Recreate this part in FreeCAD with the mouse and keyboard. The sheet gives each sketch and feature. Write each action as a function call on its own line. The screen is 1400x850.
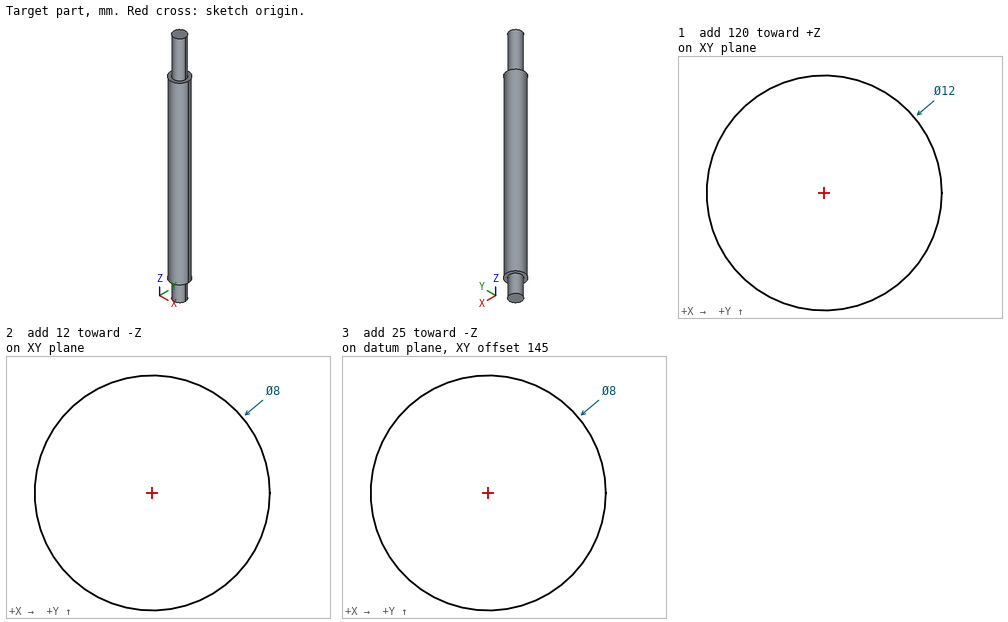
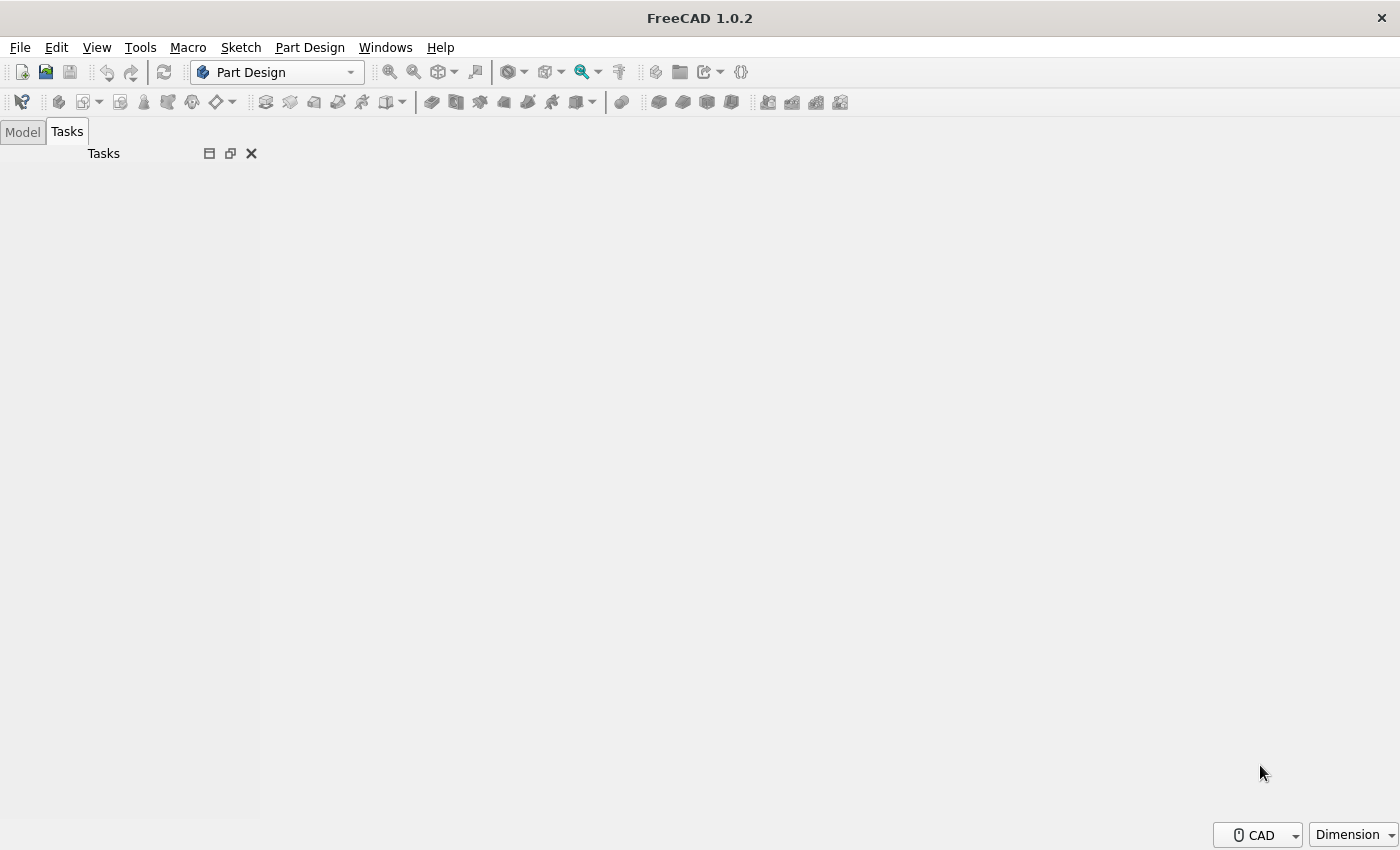
click(22, 72)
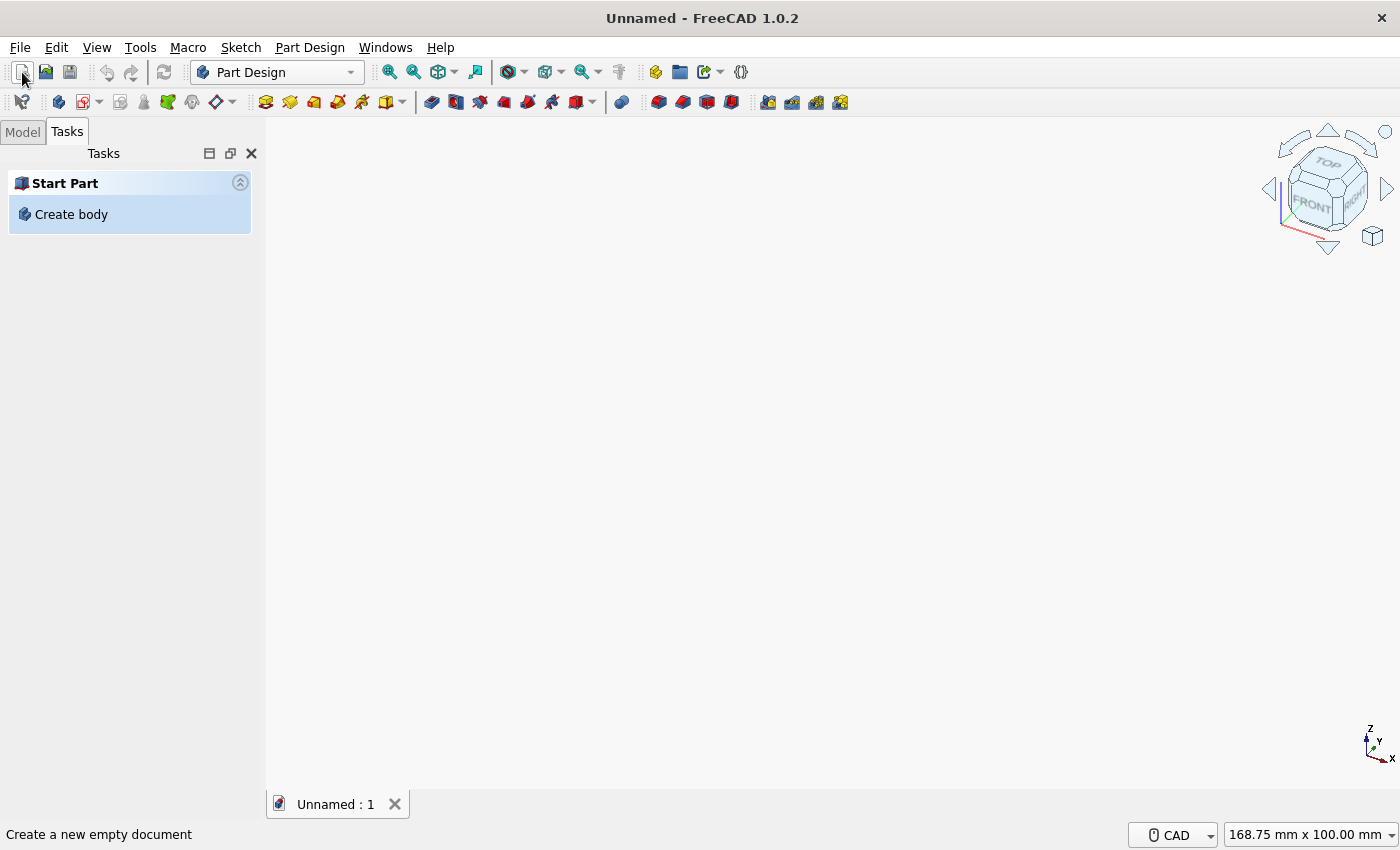
click(84, 102)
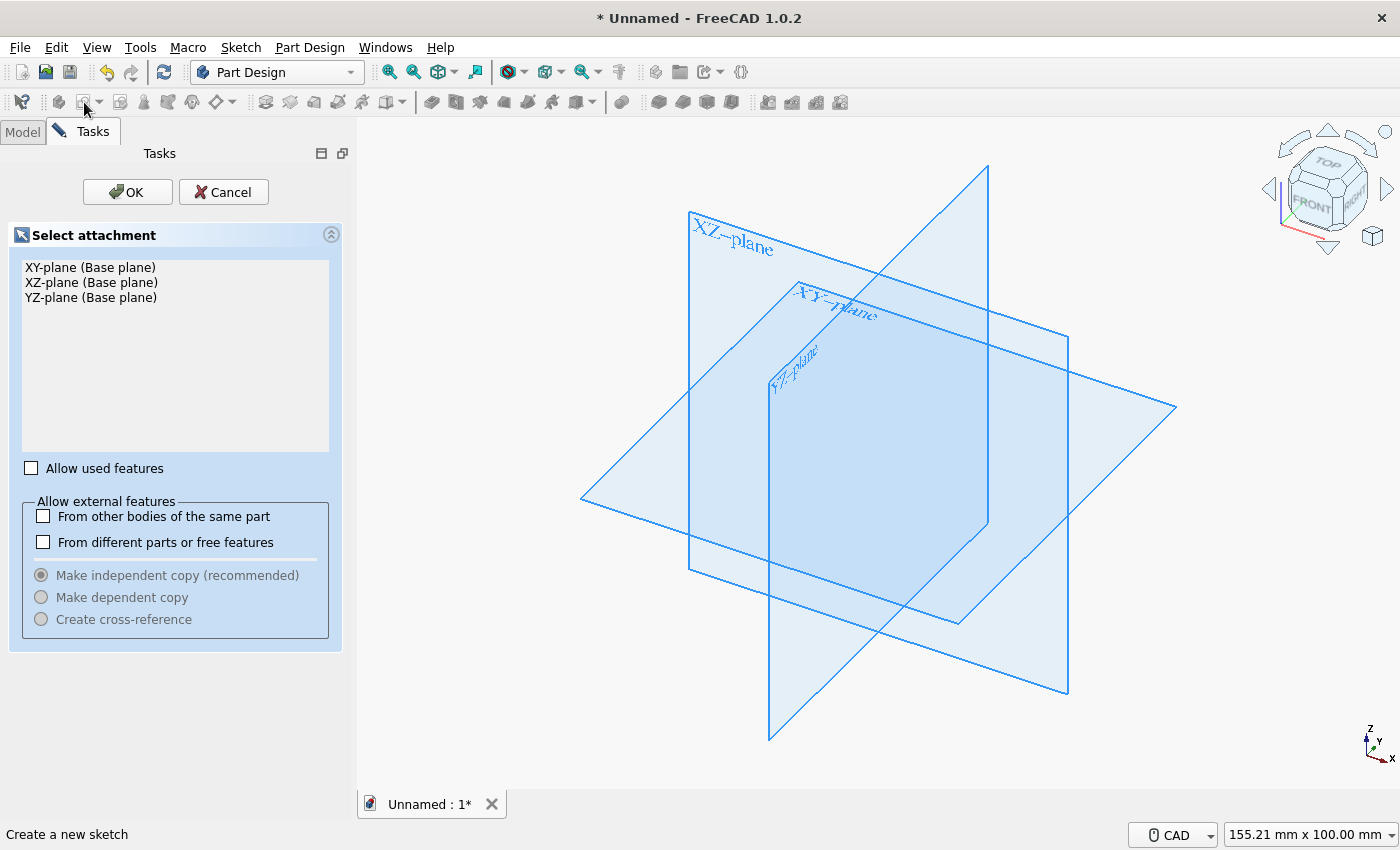
click(82, 268)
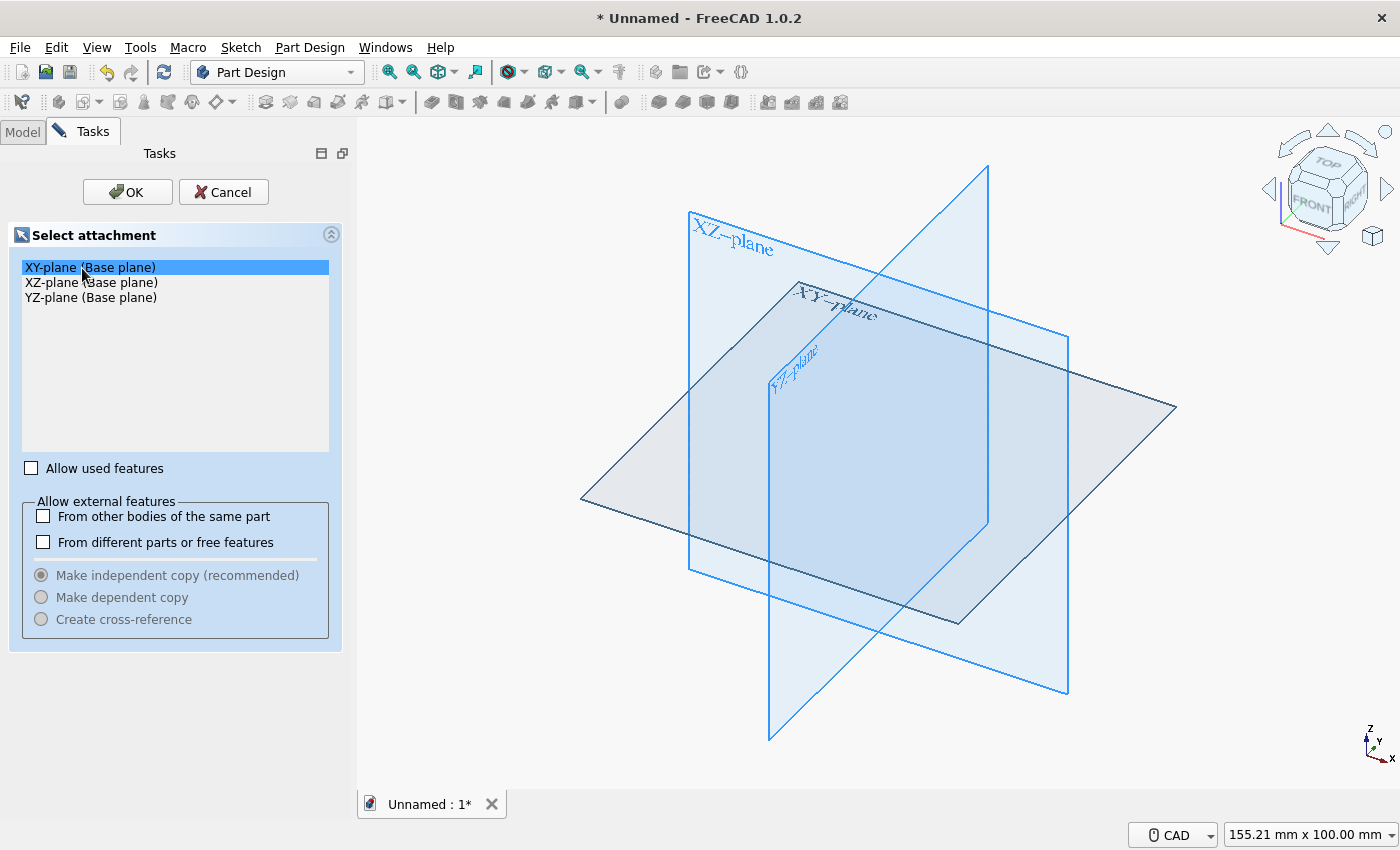
click(128, 192)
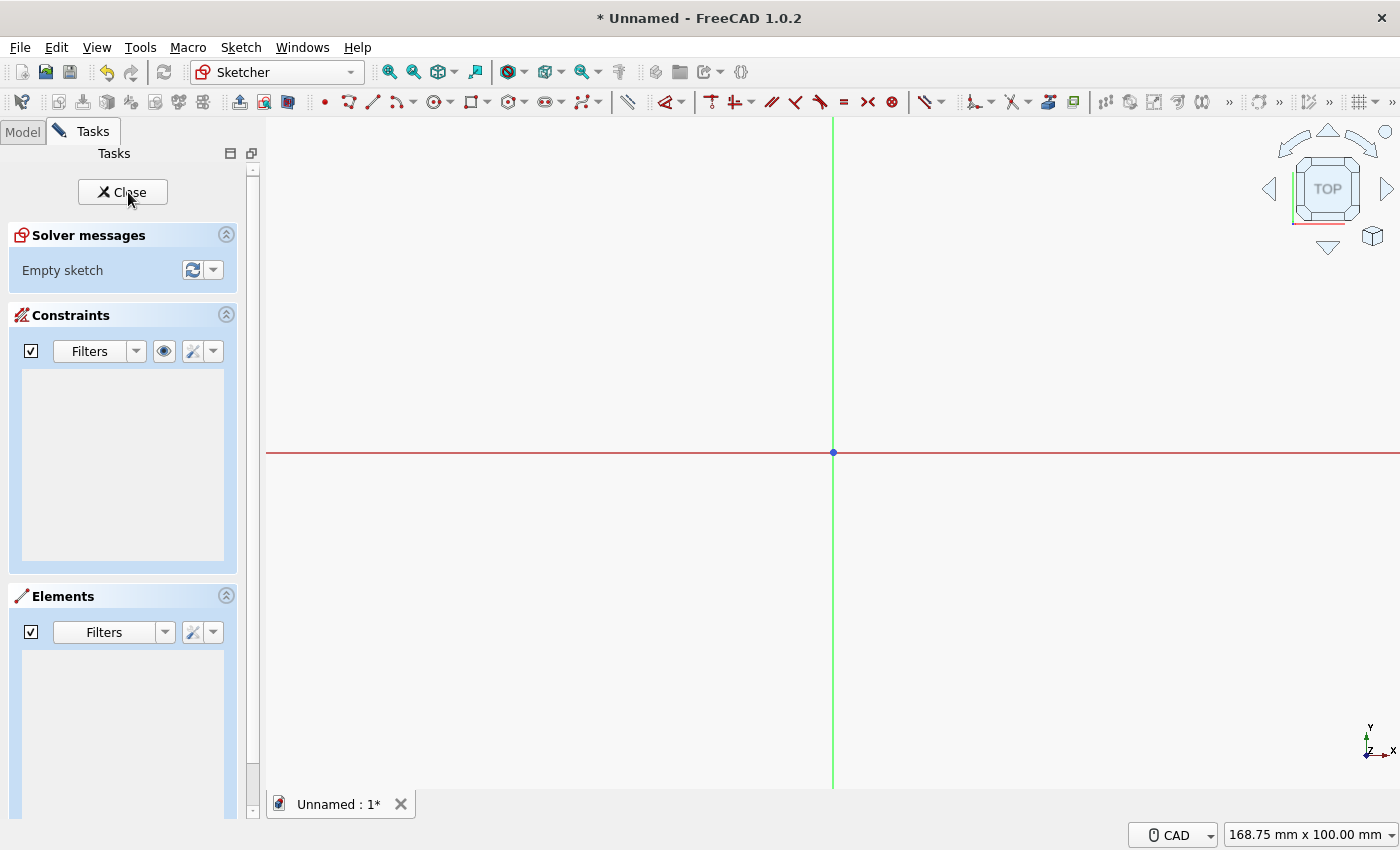
scroll(850, 453, up, 8)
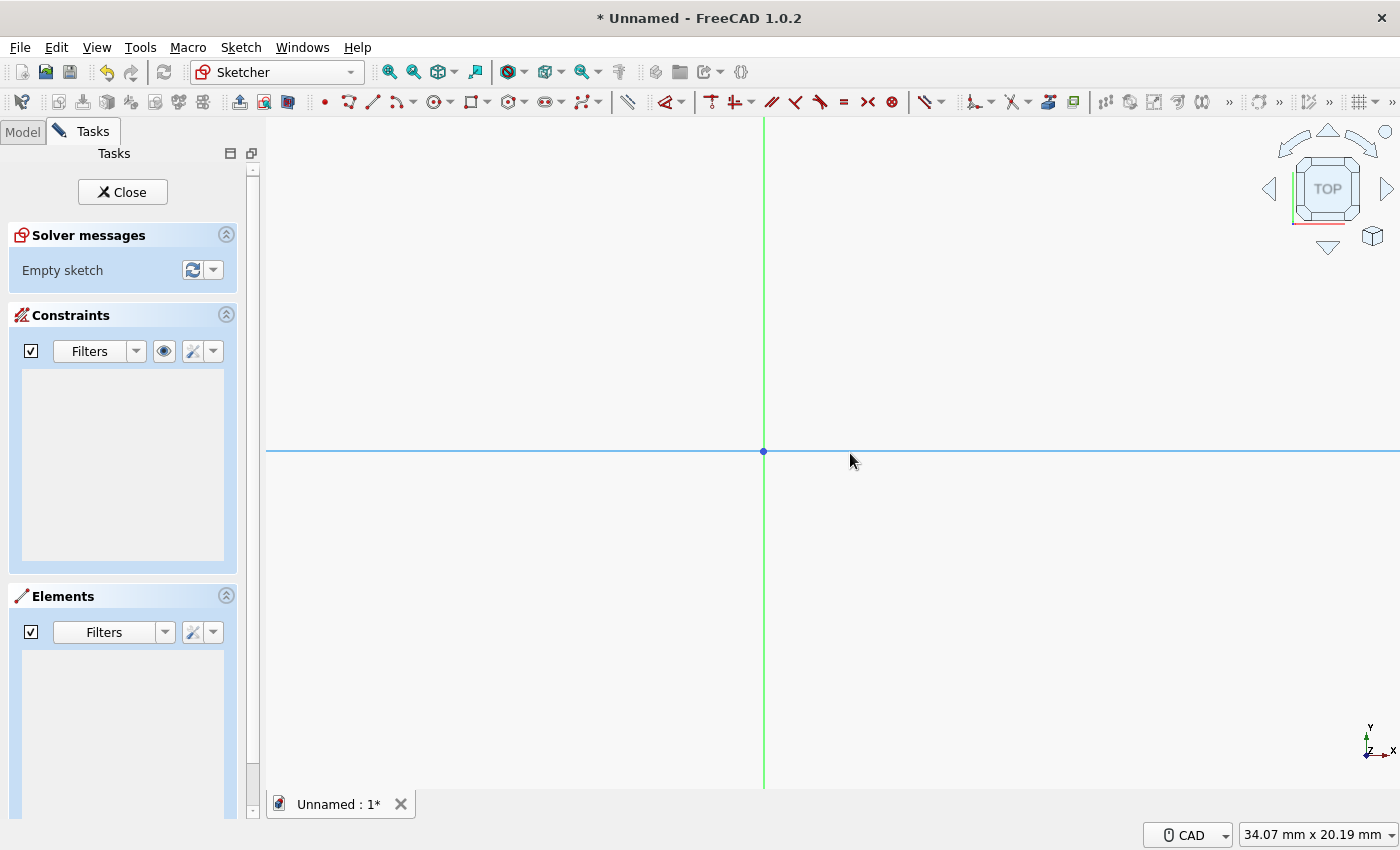
key(g)
key(c)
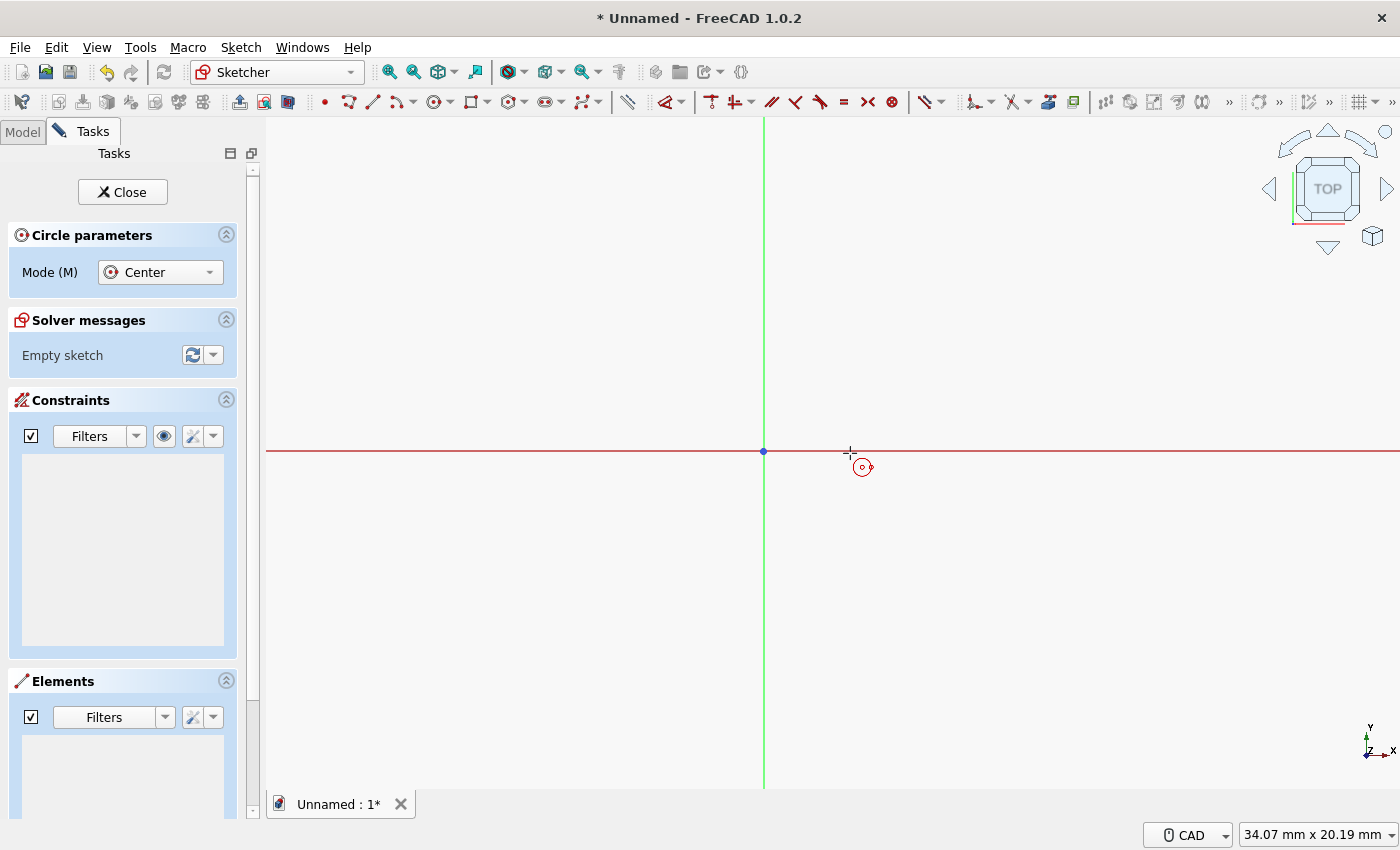
click(764, 451)
click(905, 310)
key(Escape)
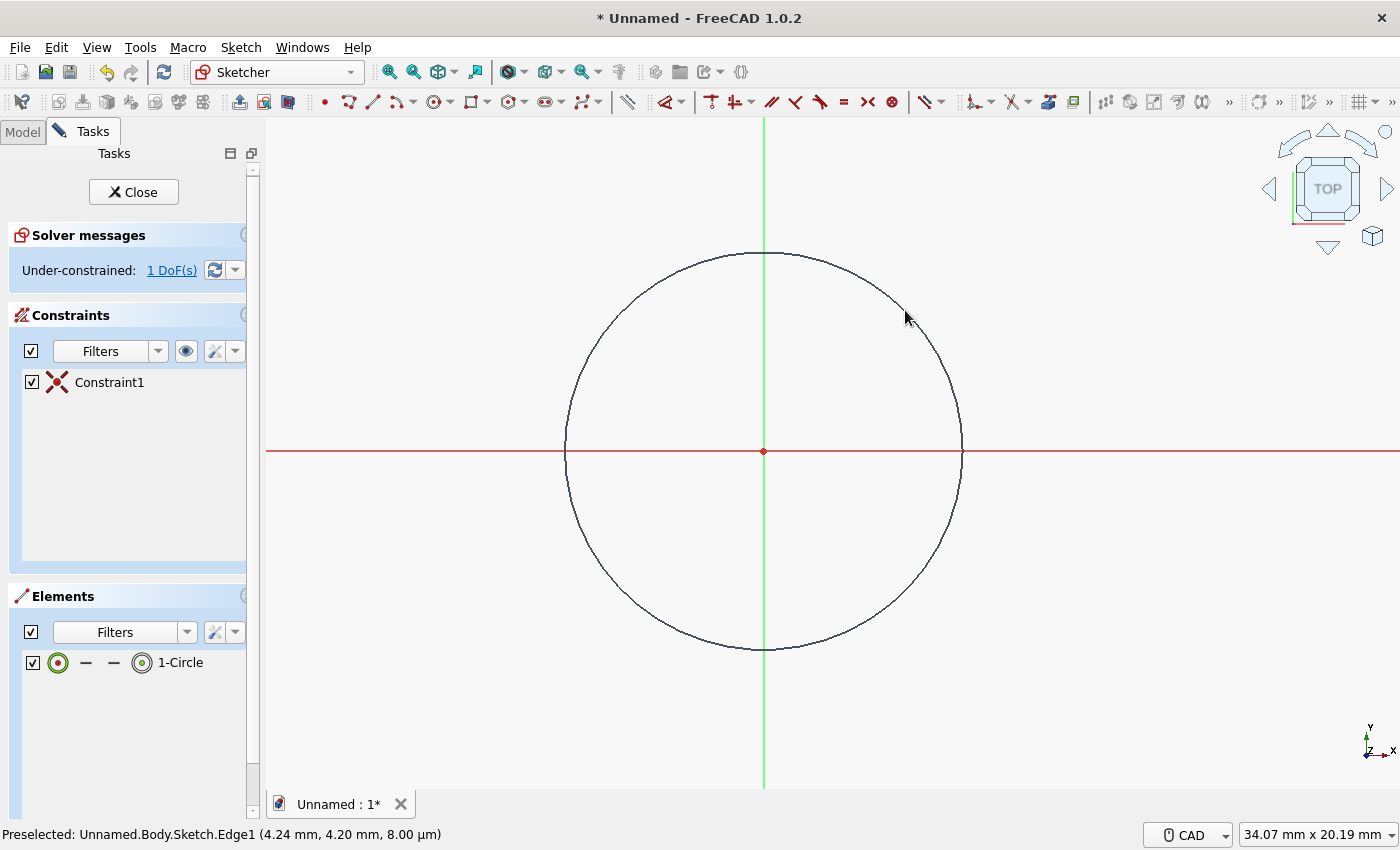
click(666, 102)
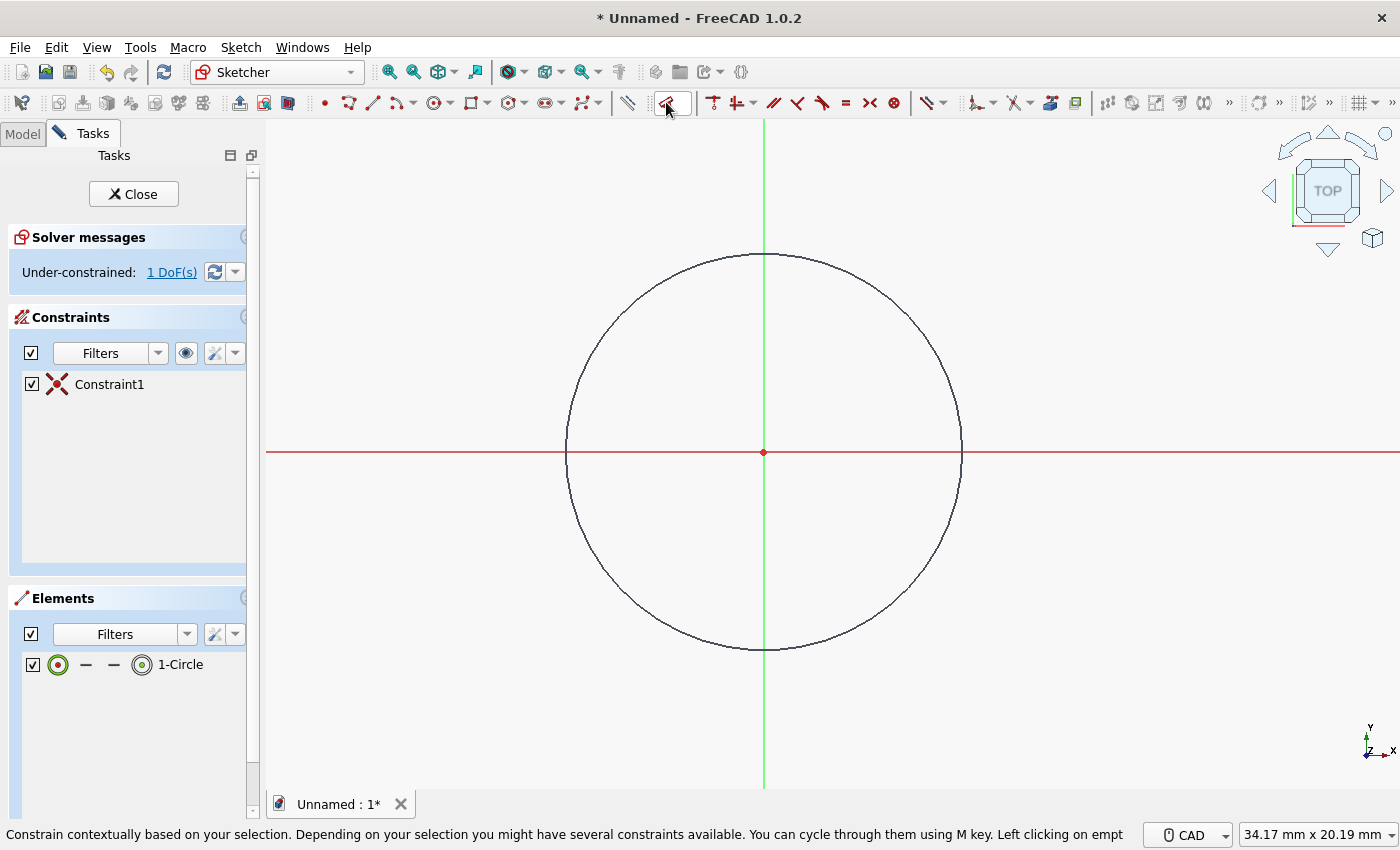
click(904, 311)
click(927, 288)